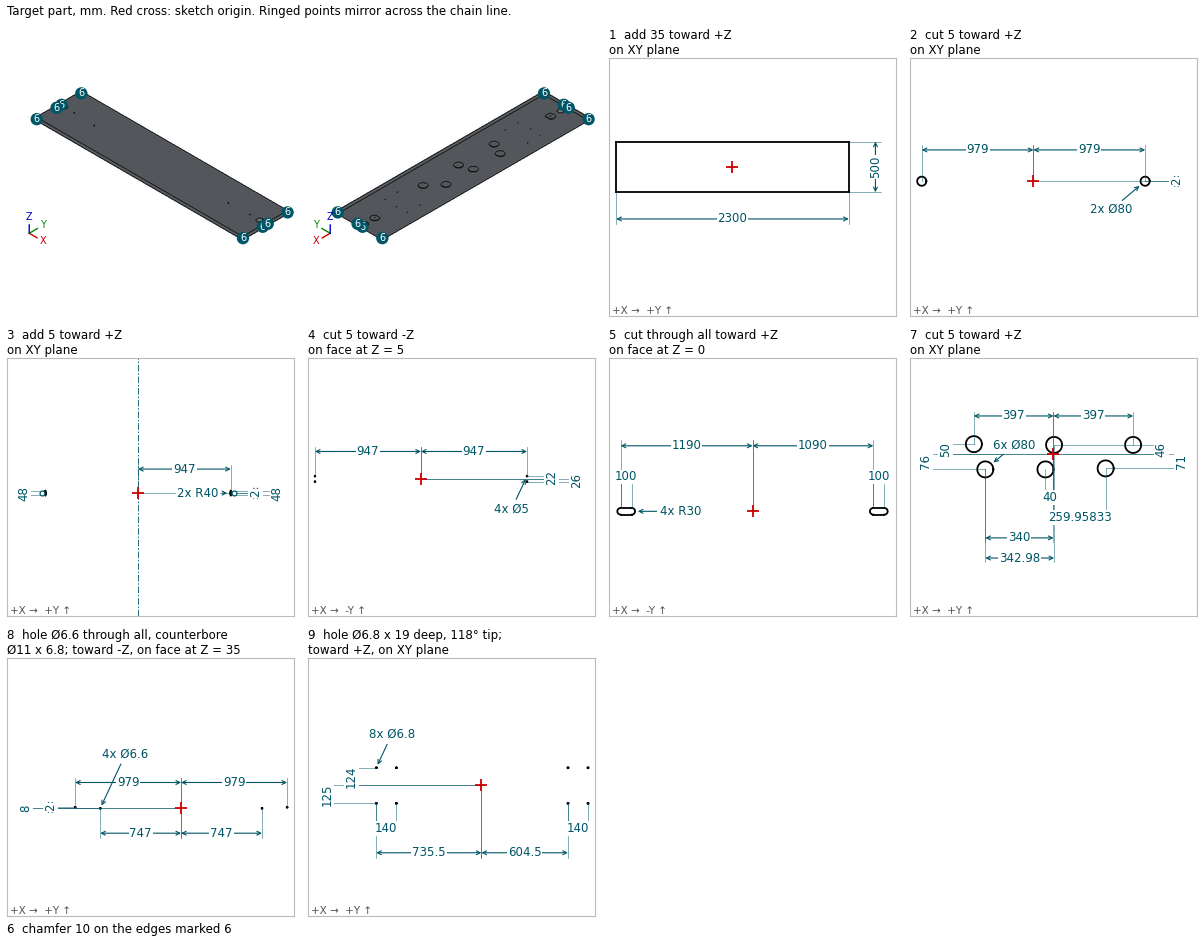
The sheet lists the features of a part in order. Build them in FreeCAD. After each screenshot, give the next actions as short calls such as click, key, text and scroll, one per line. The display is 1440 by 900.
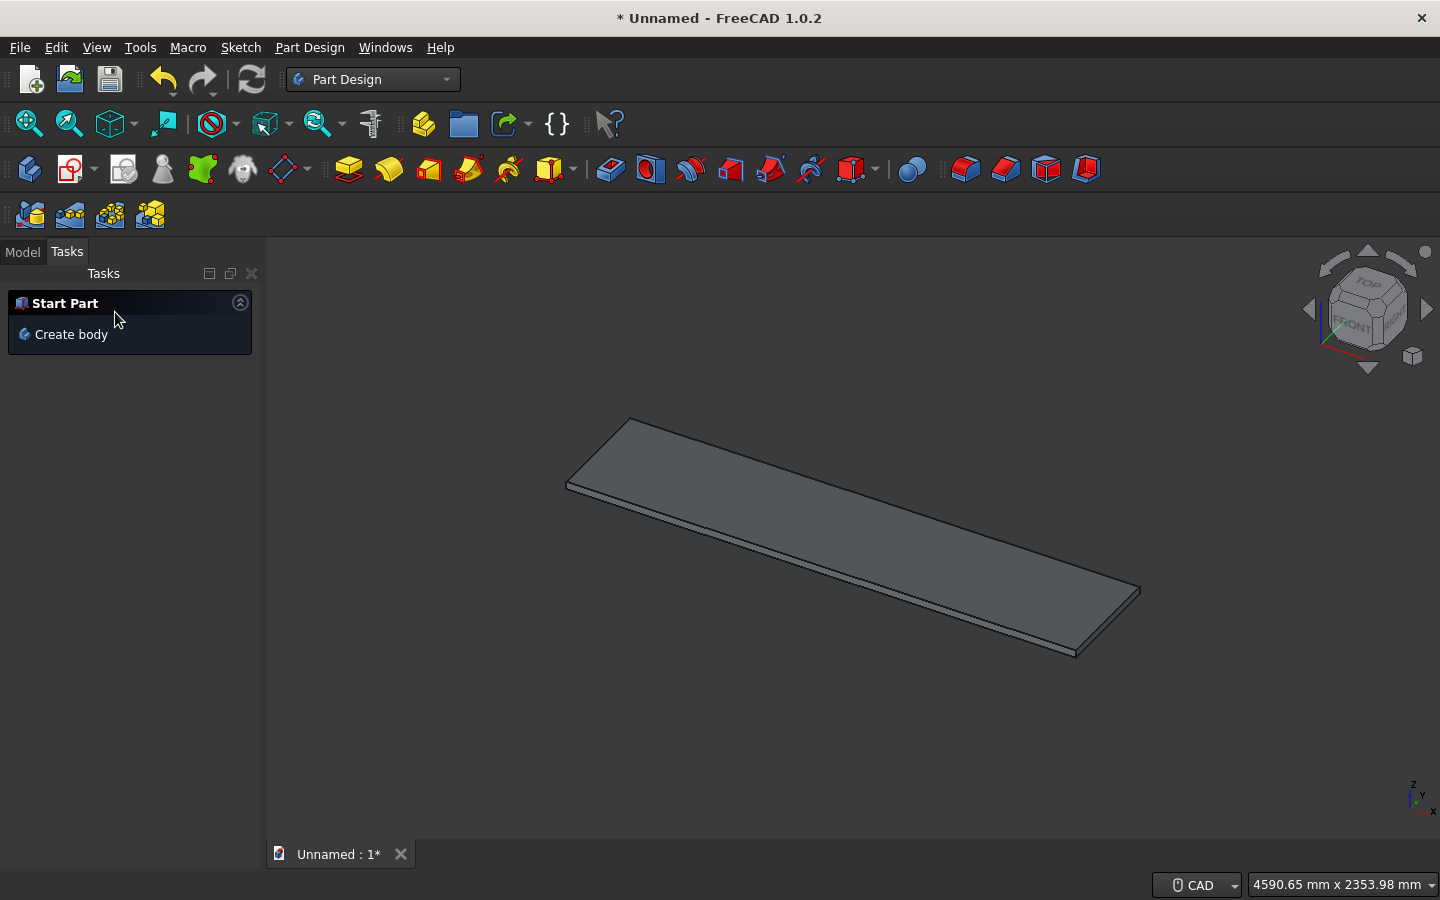
click(70, 170)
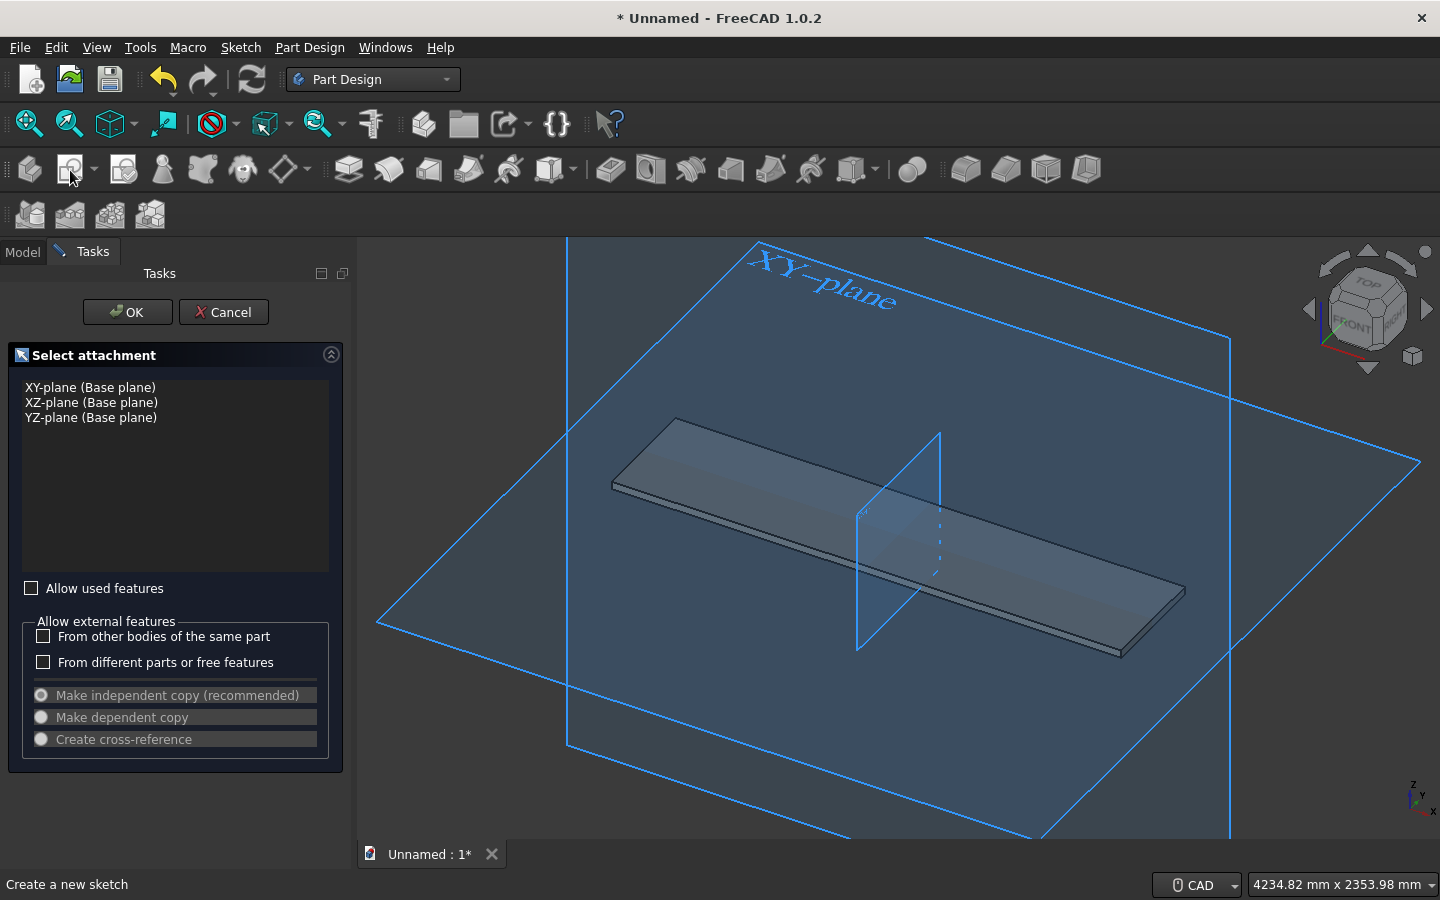
click(82, 388)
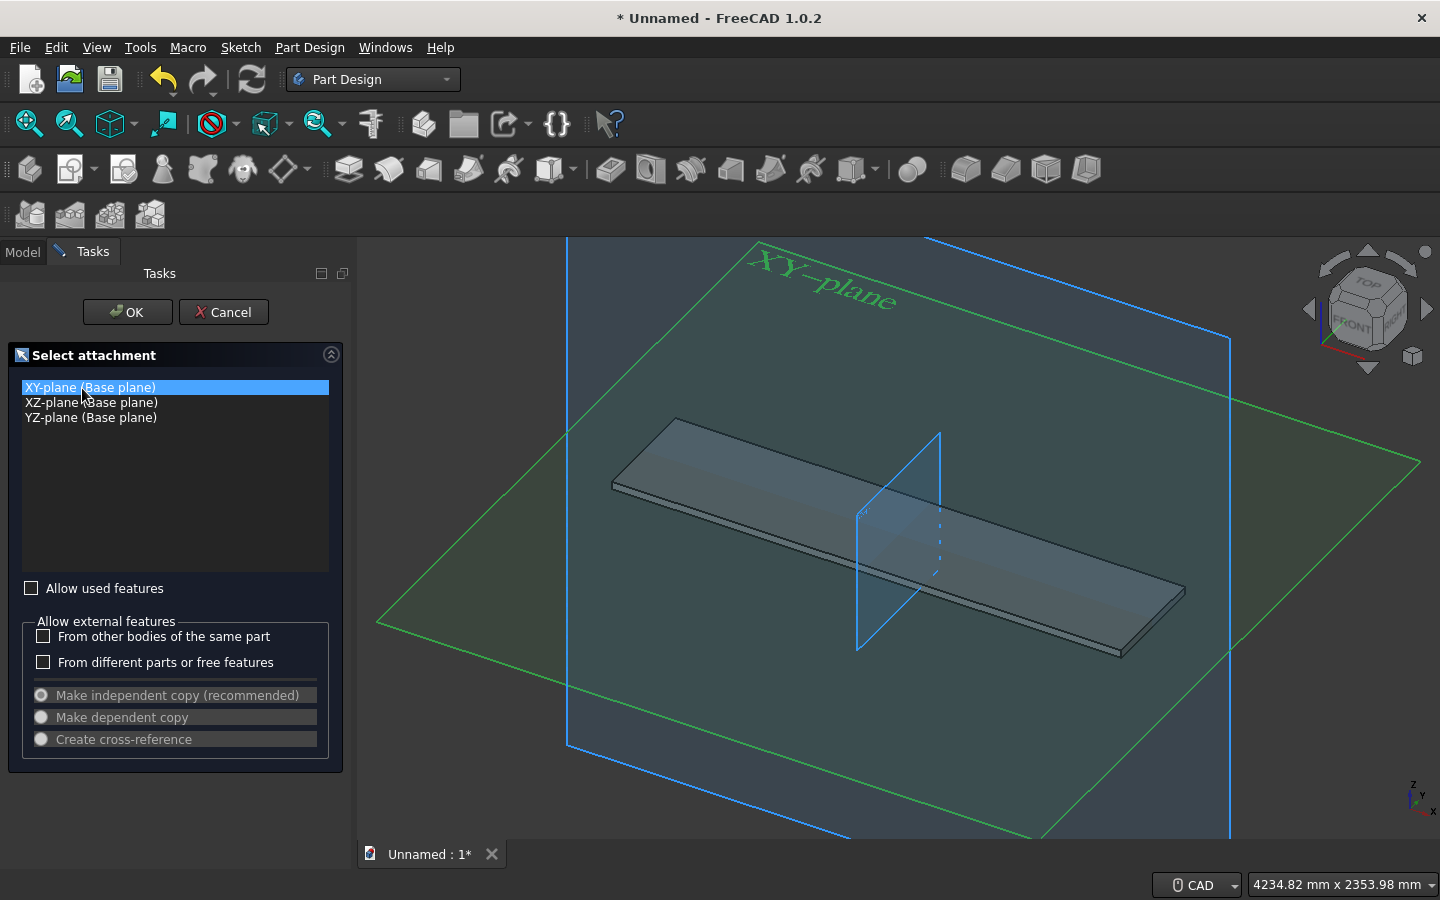
click(128, 312)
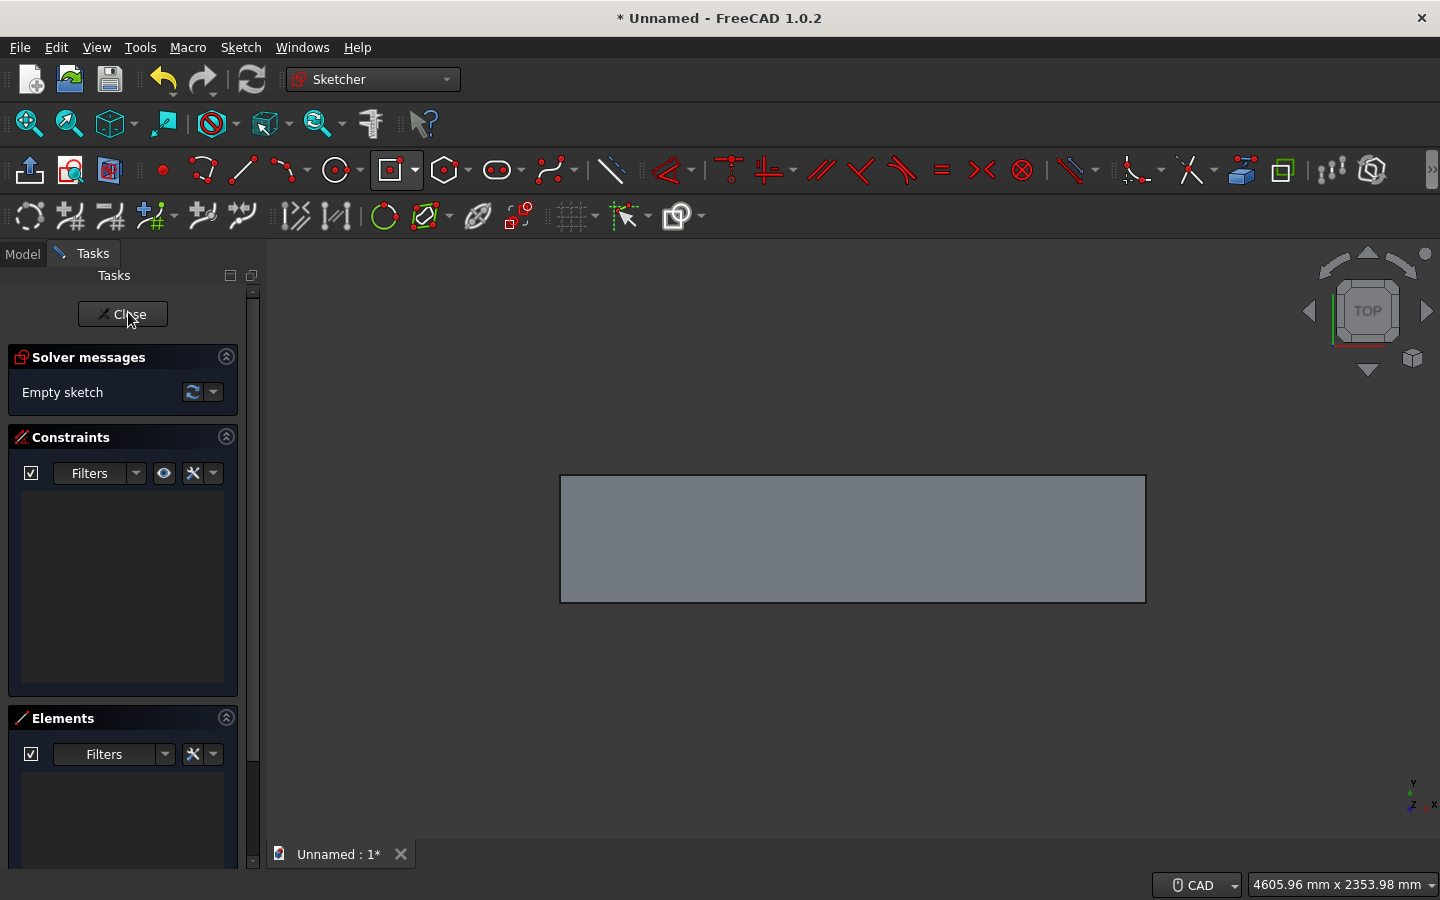
click(110, 170)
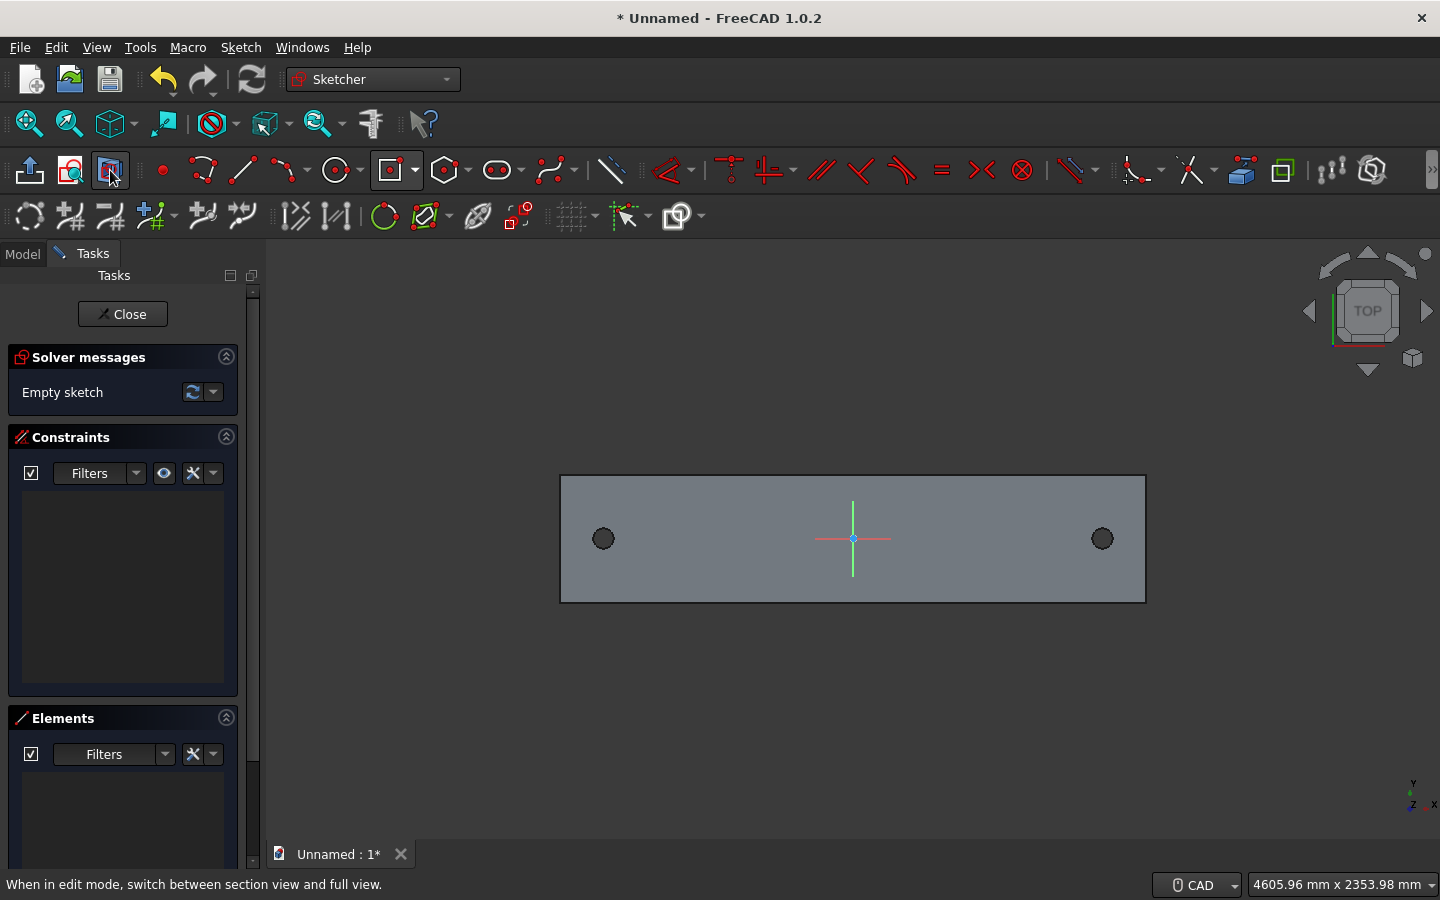
scroll(992, 537, up, 2)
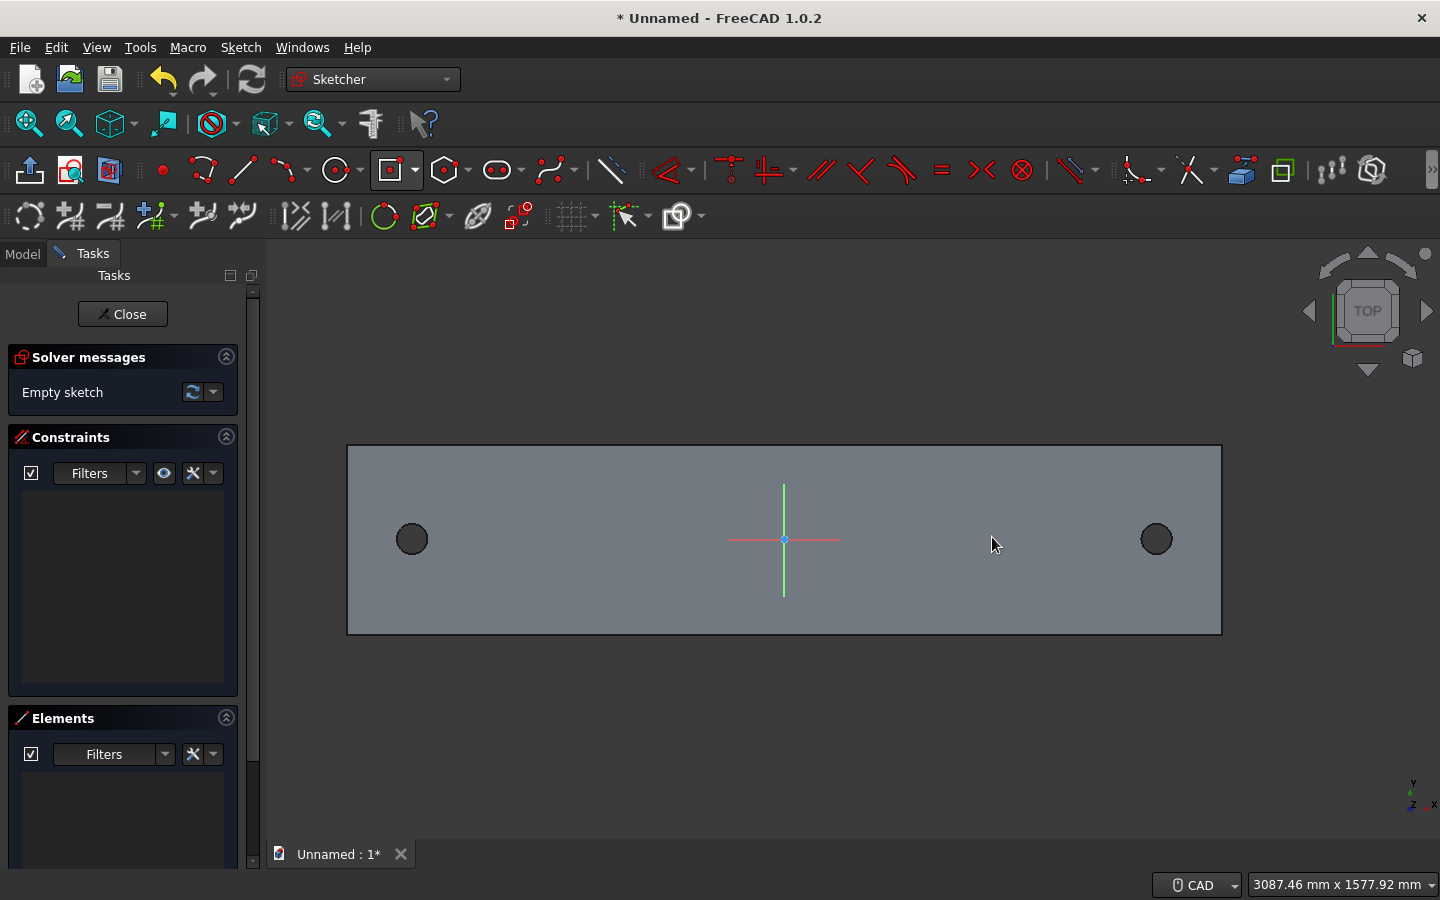
key(g)
key(l)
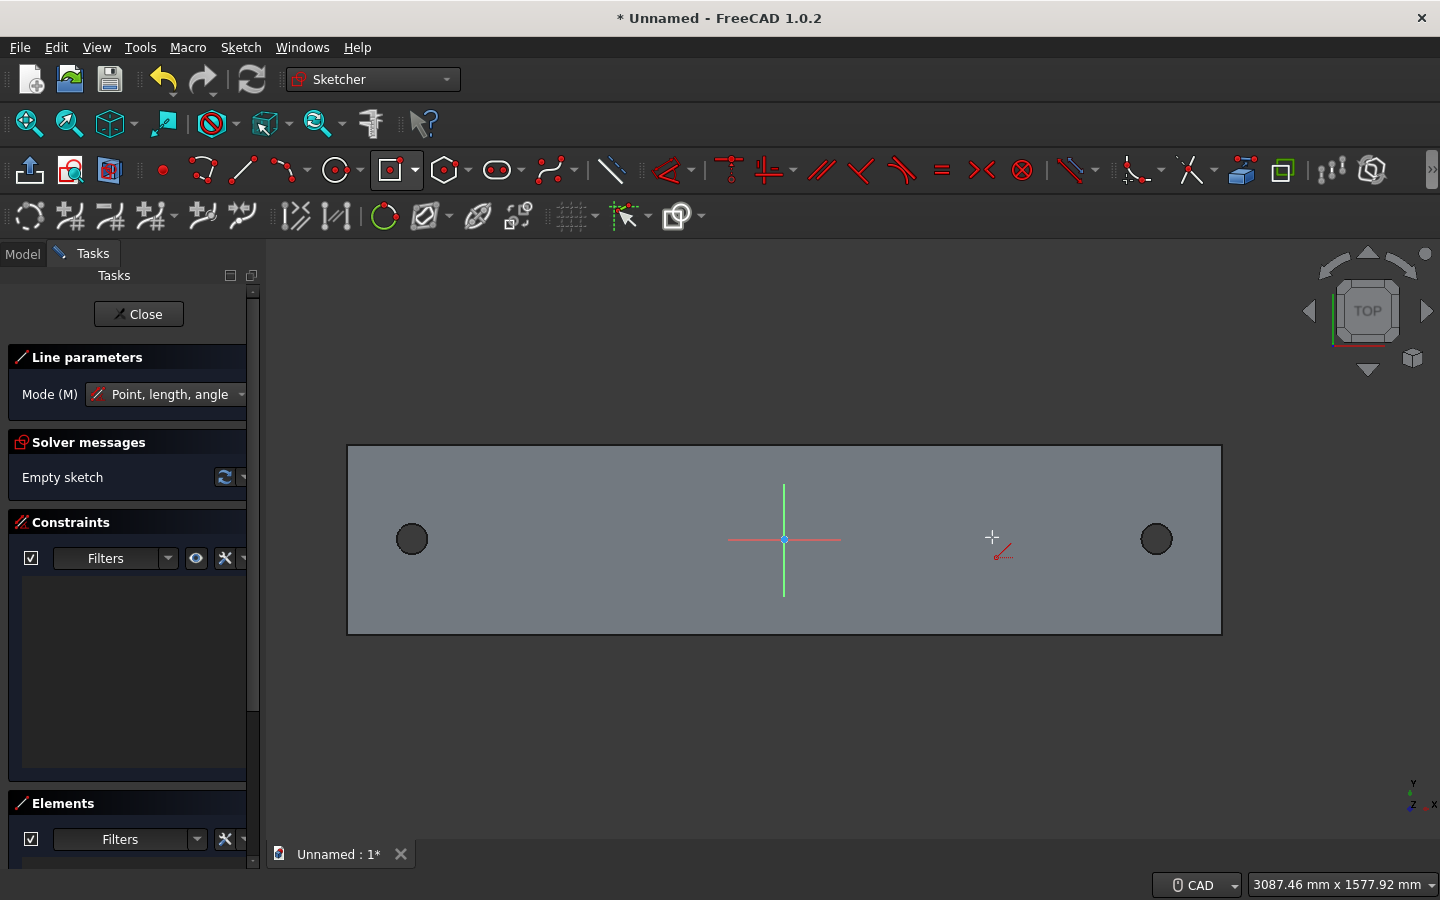
scroll(1144, 530, up, 3)